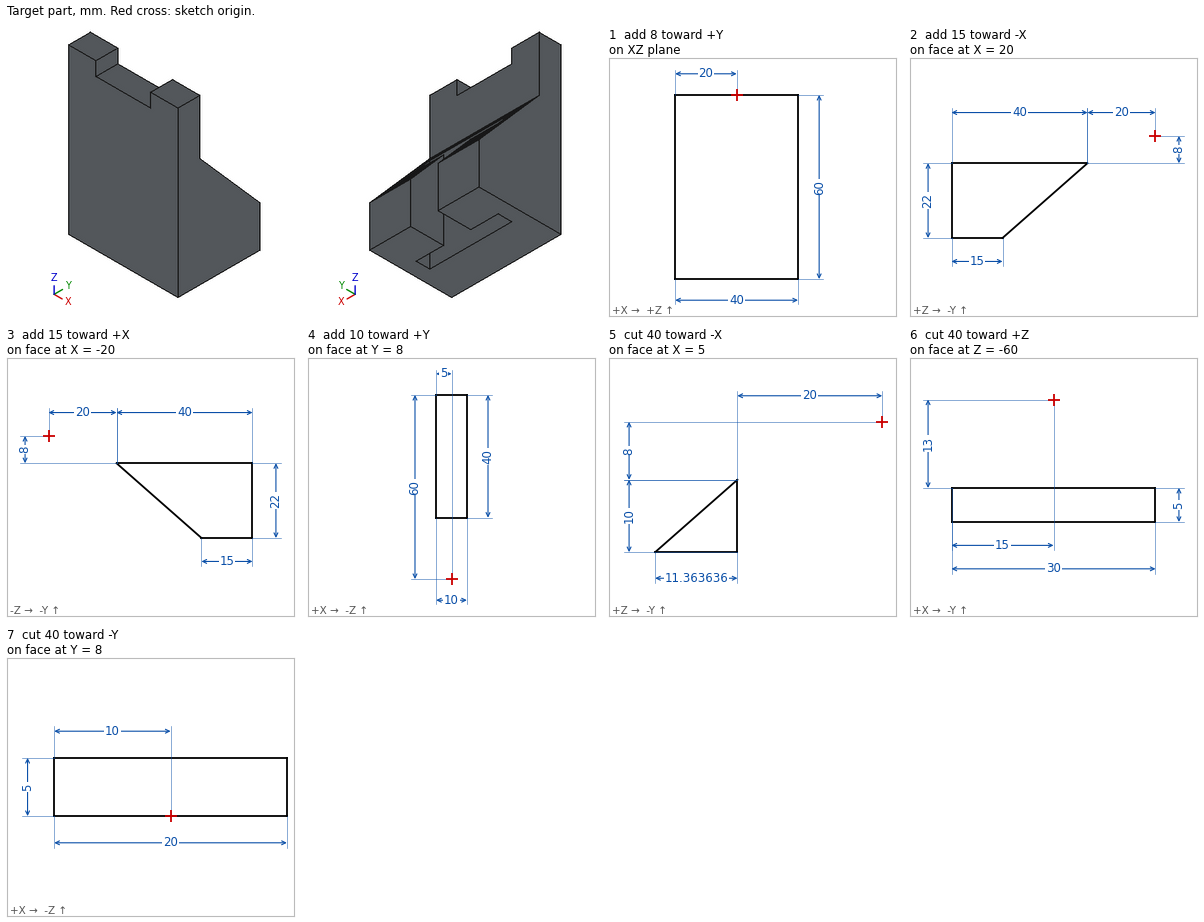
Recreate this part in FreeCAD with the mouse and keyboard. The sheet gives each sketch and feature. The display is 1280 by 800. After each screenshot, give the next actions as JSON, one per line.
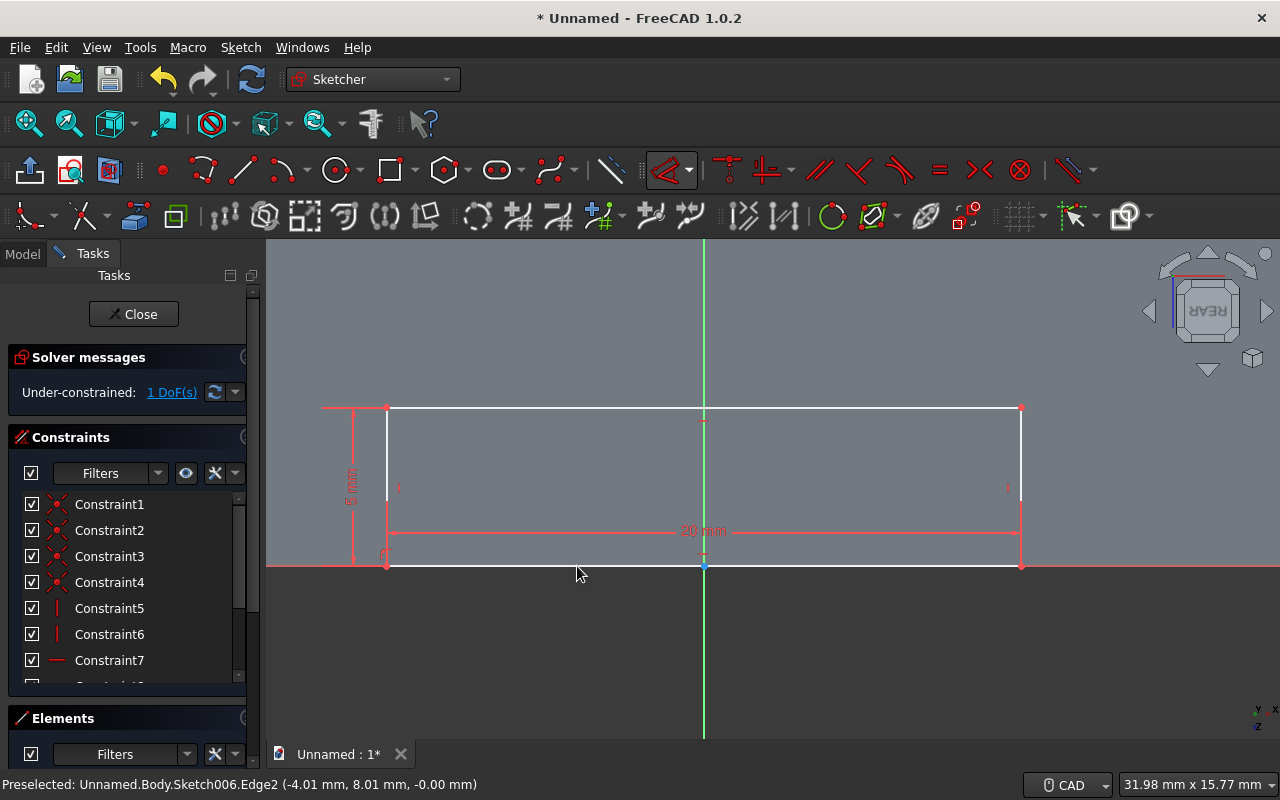
{"action": "left_click", "coordinate": [387, 408]}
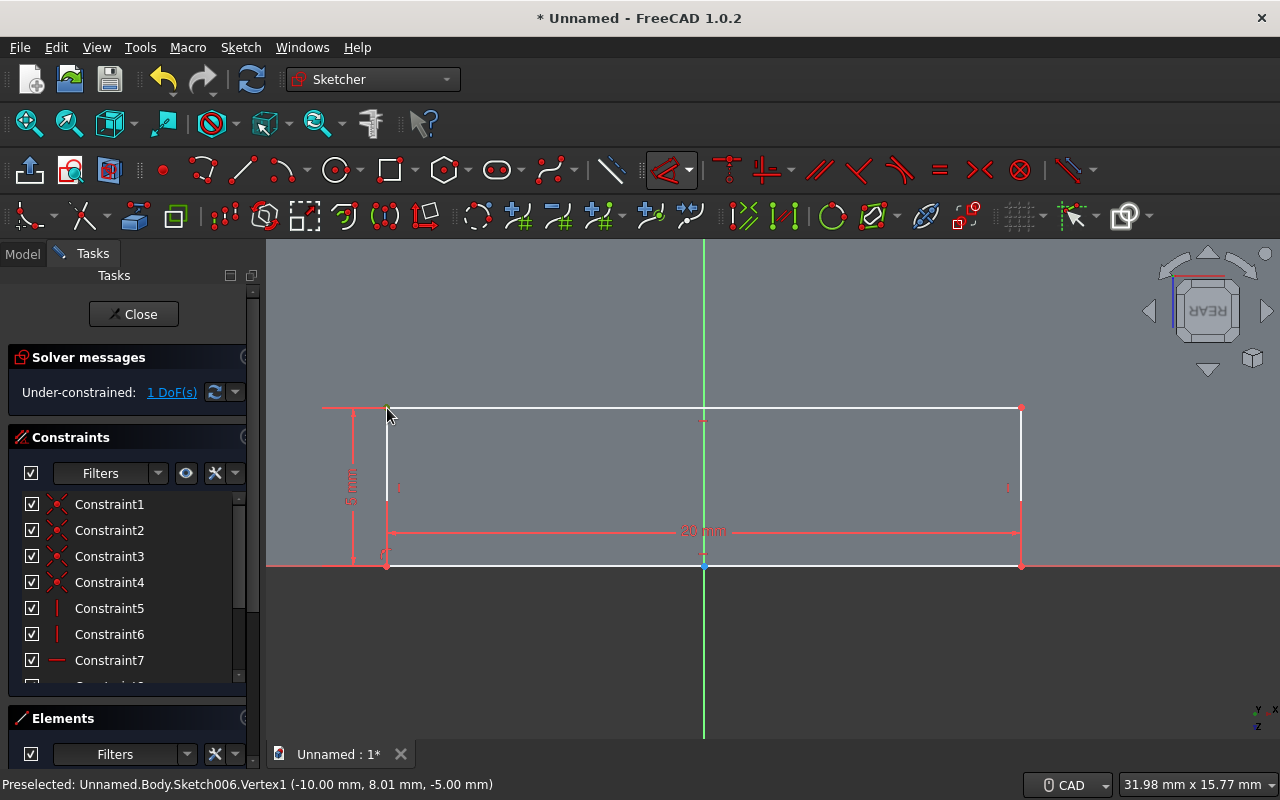
{"action": "left_click", "coordinate": [692, 170]}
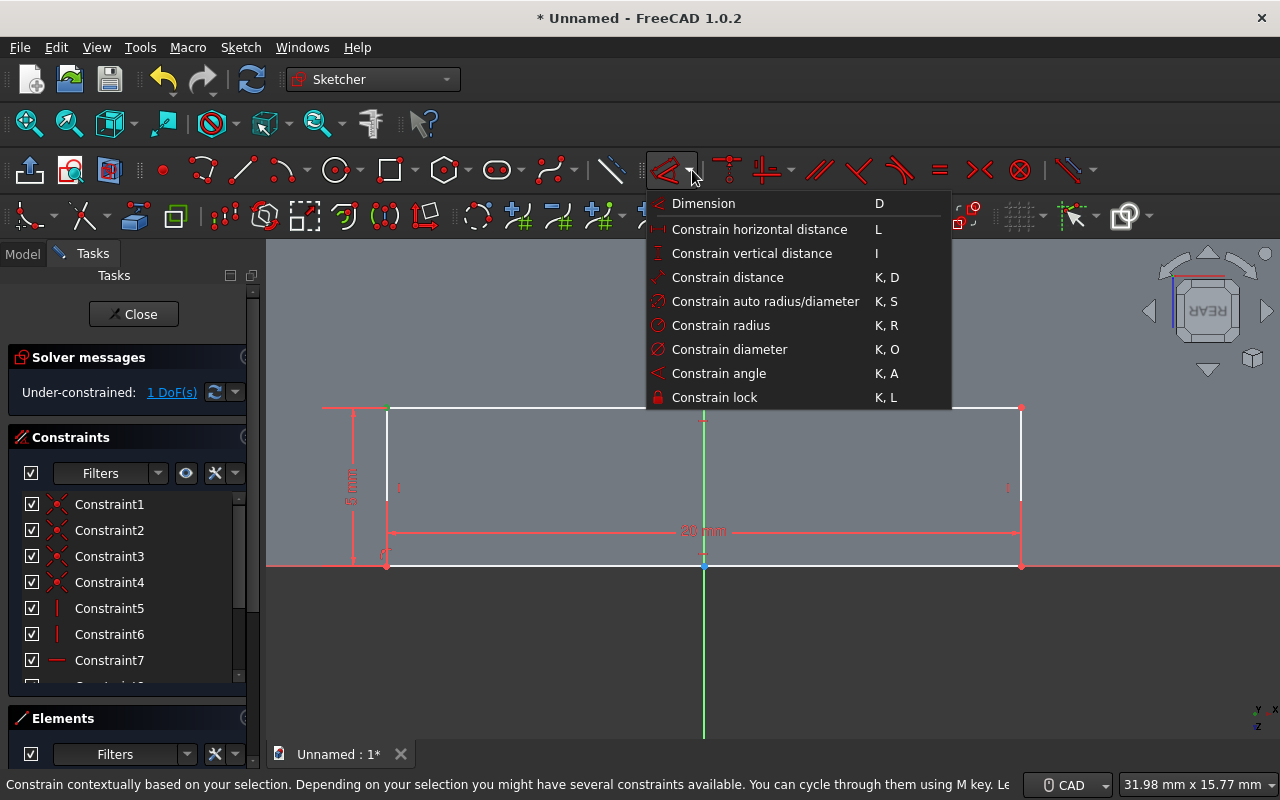
{"action": "left_click", "coordinate": [799, 229]}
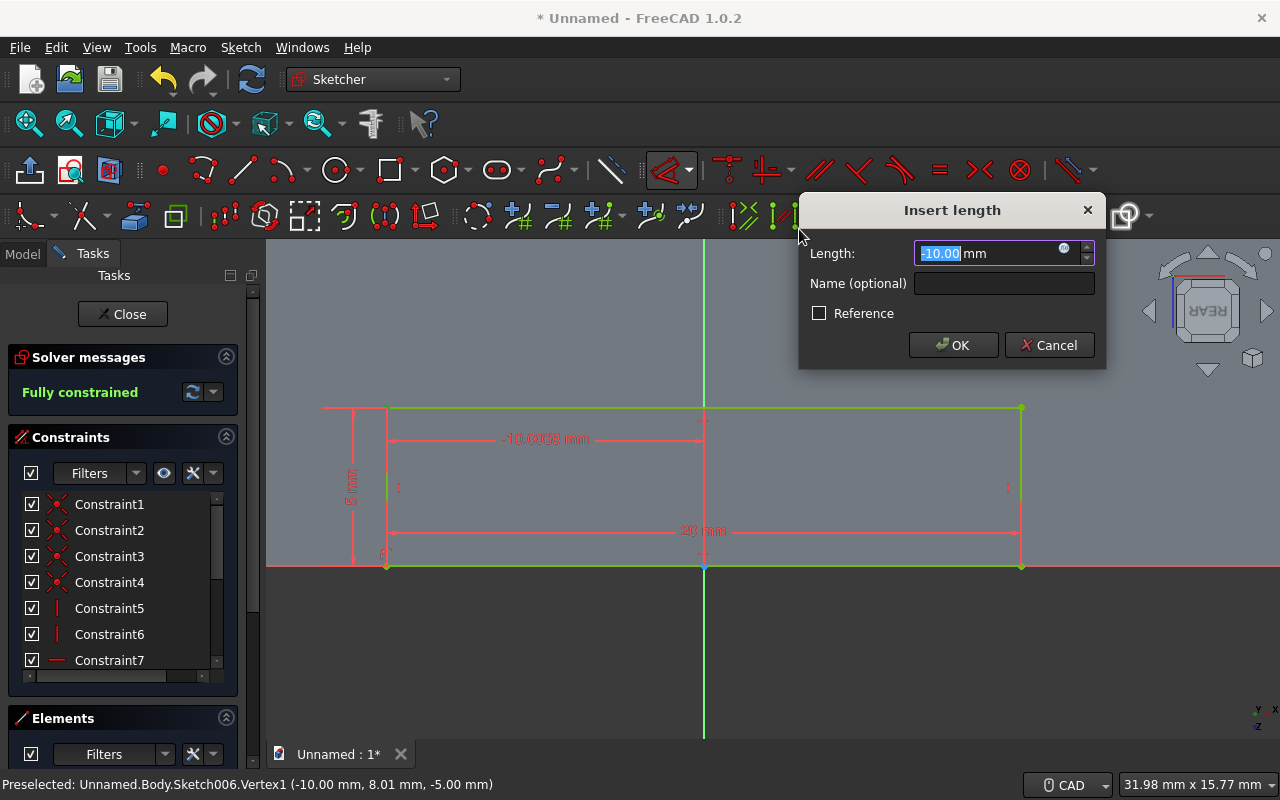
{"action": "type", "text": "-10"}
{"action": "key", "text": "Return"}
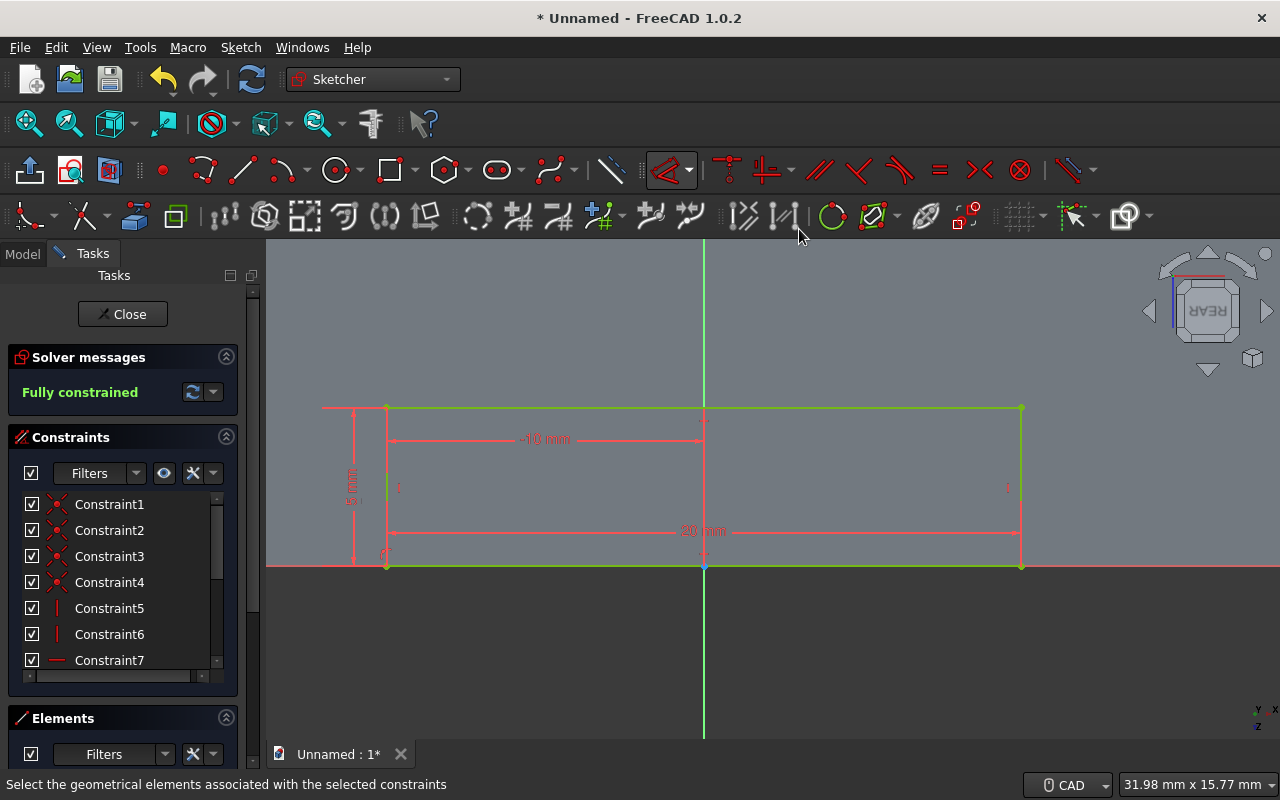
{"action": "left_click", "coordinate": [123, 314]}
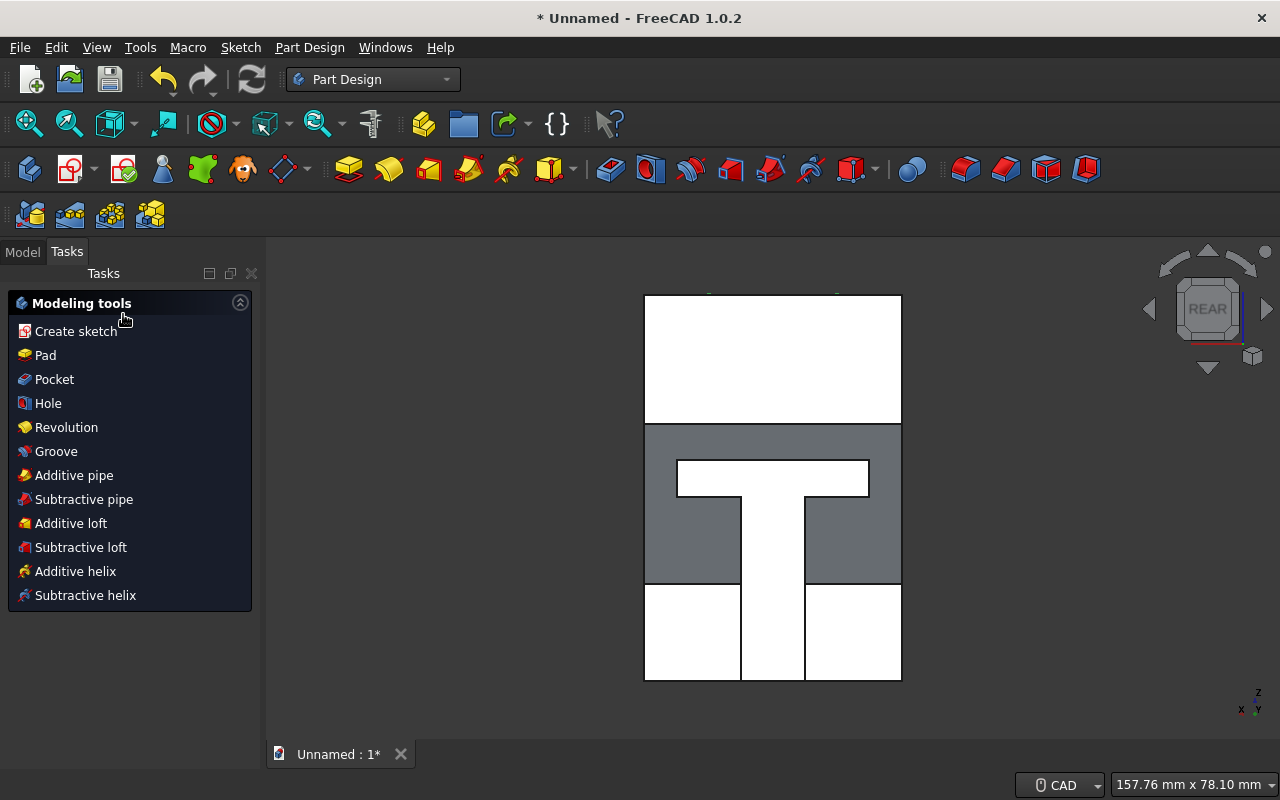
{"action": "left_click", "coordinate": [612, 170]}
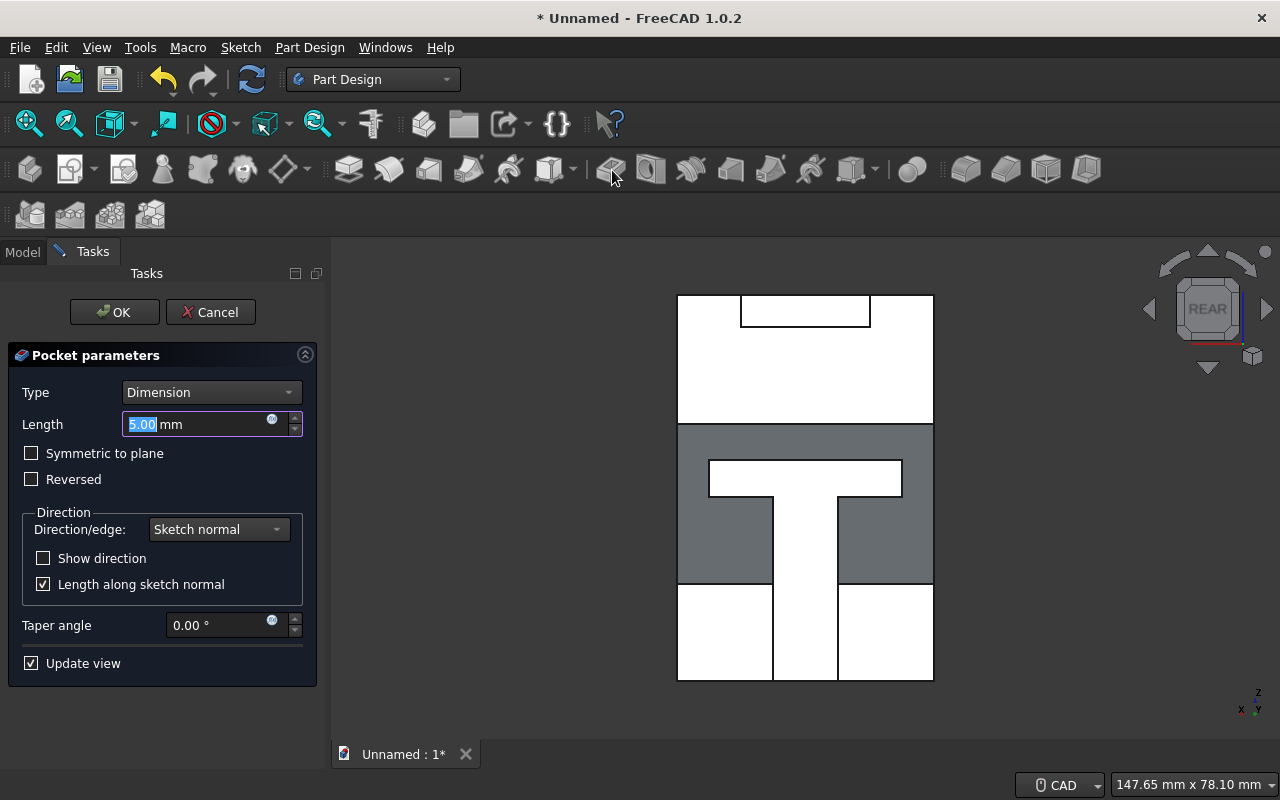
{"action": "type", "text": "40"}
{"action": "key", "text": "Tab"}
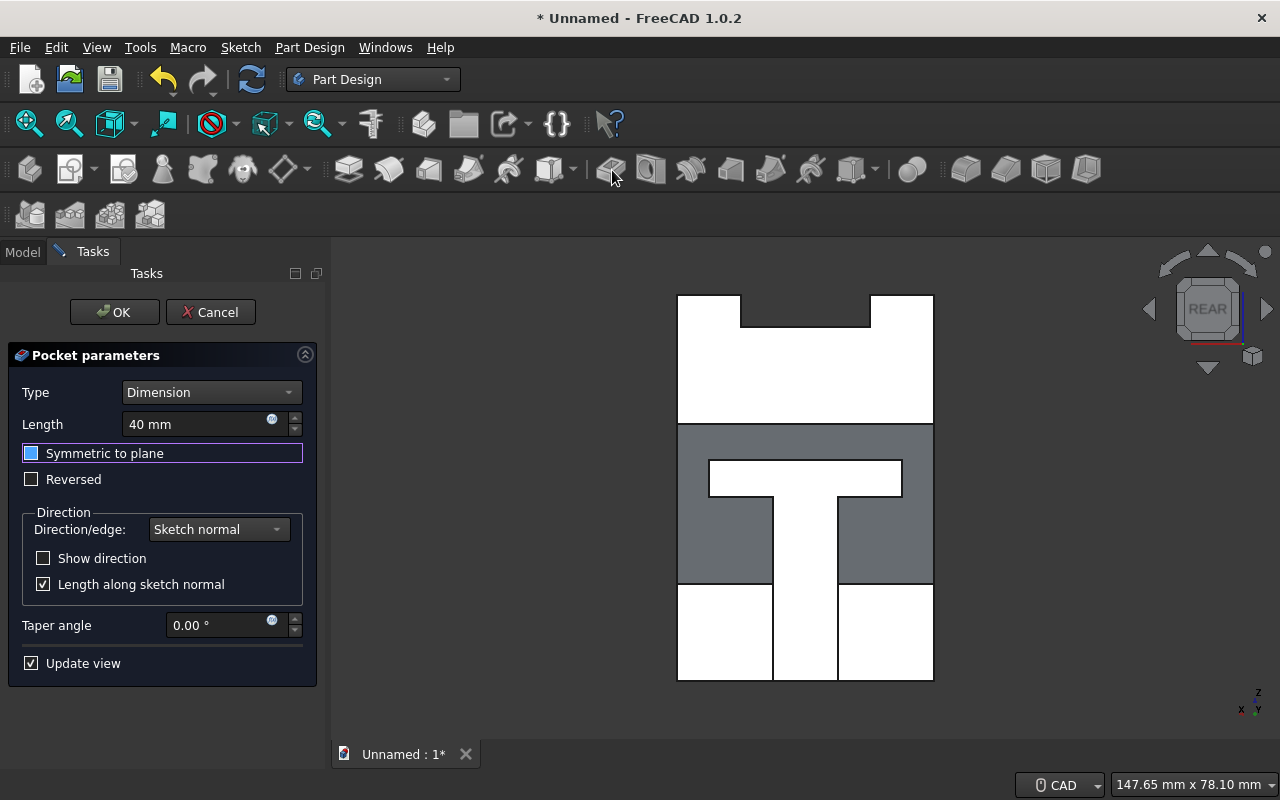
{"action": "left_click", "coordinate": [115, 312]}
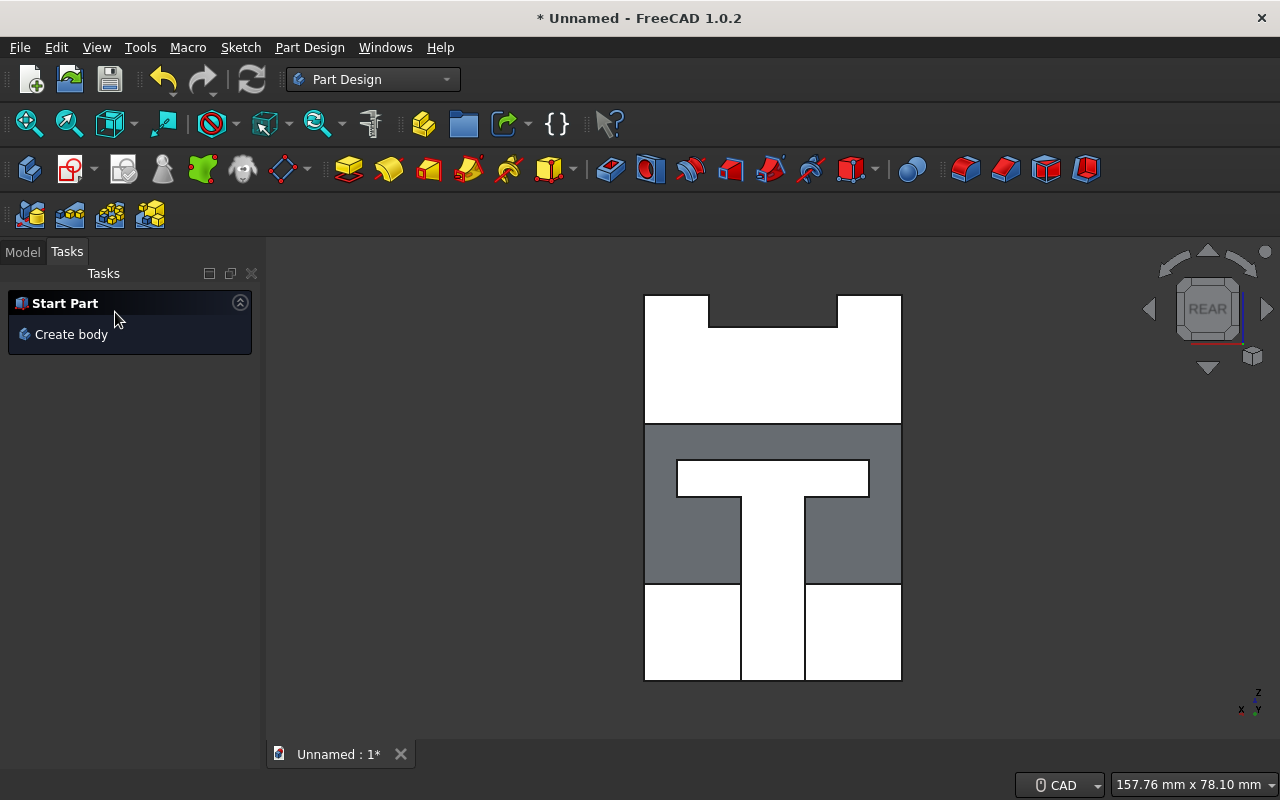
{"action": "key", "text": "0"}